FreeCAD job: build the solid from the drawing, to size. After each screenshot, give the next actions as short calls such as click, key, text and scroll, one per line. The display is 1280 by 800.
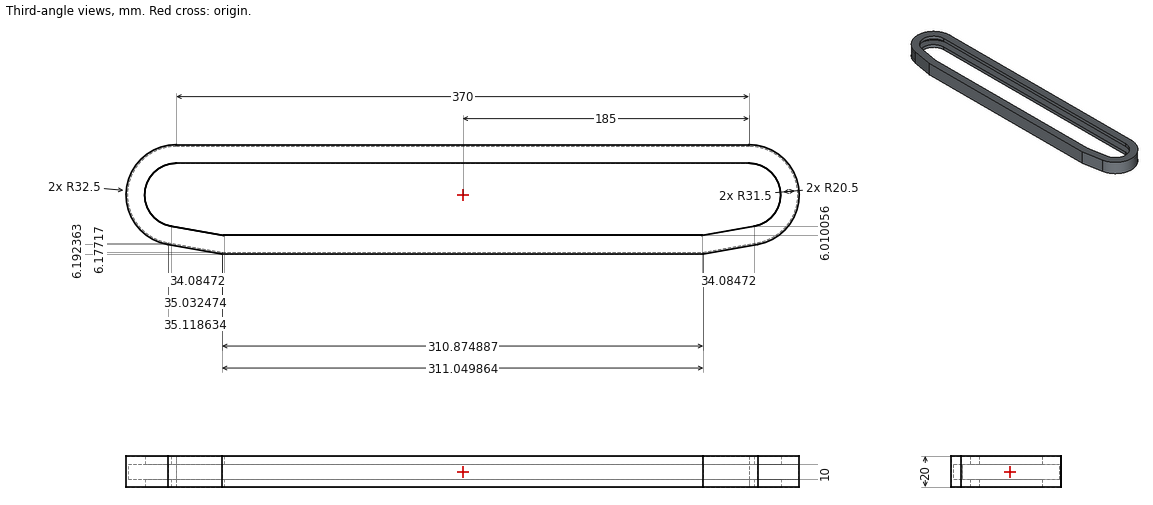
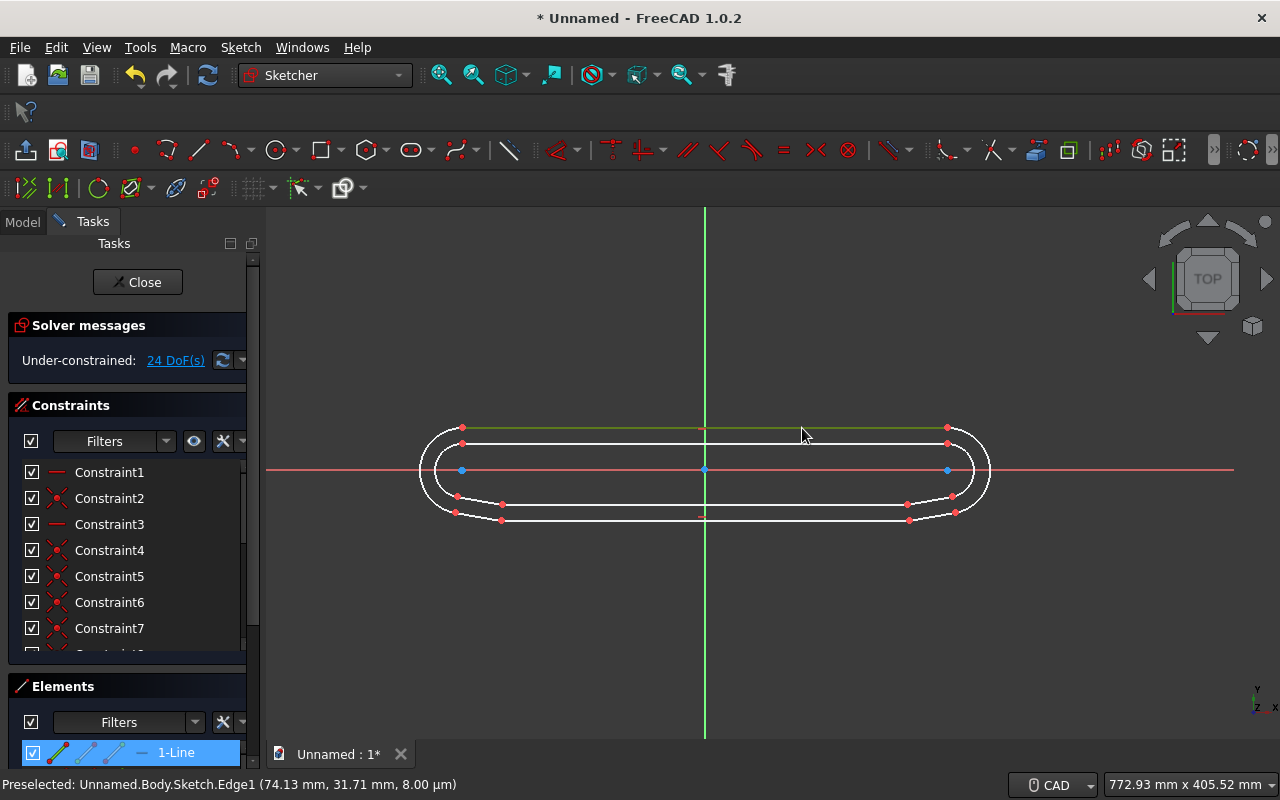
click(429, 444)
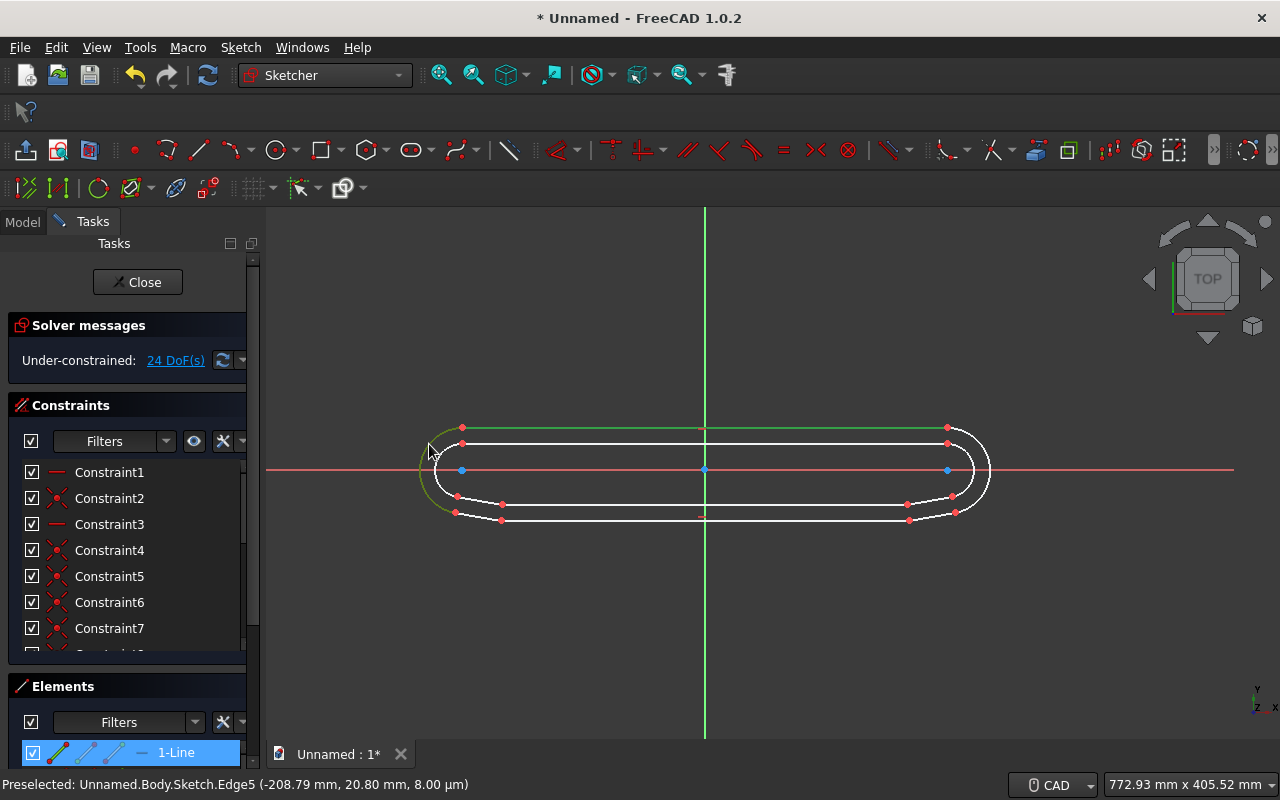
key(t)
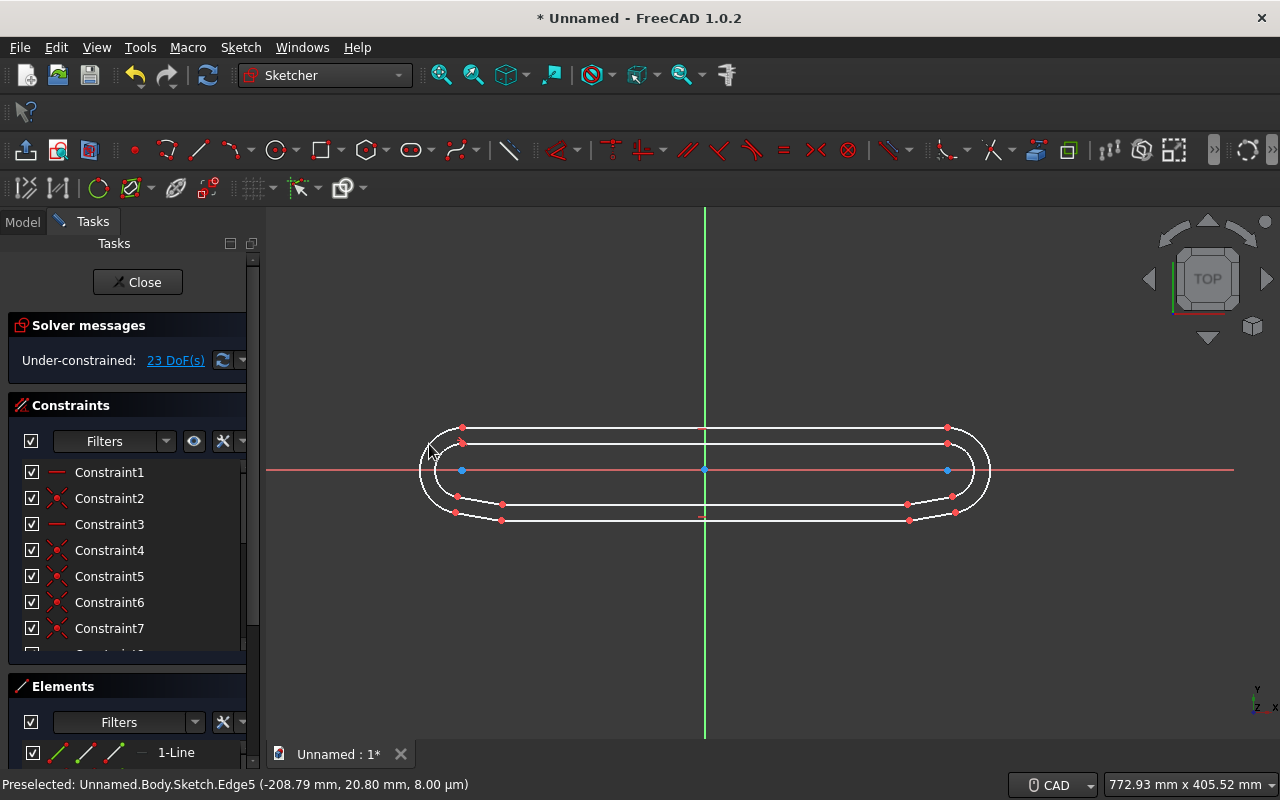
click(802, 428)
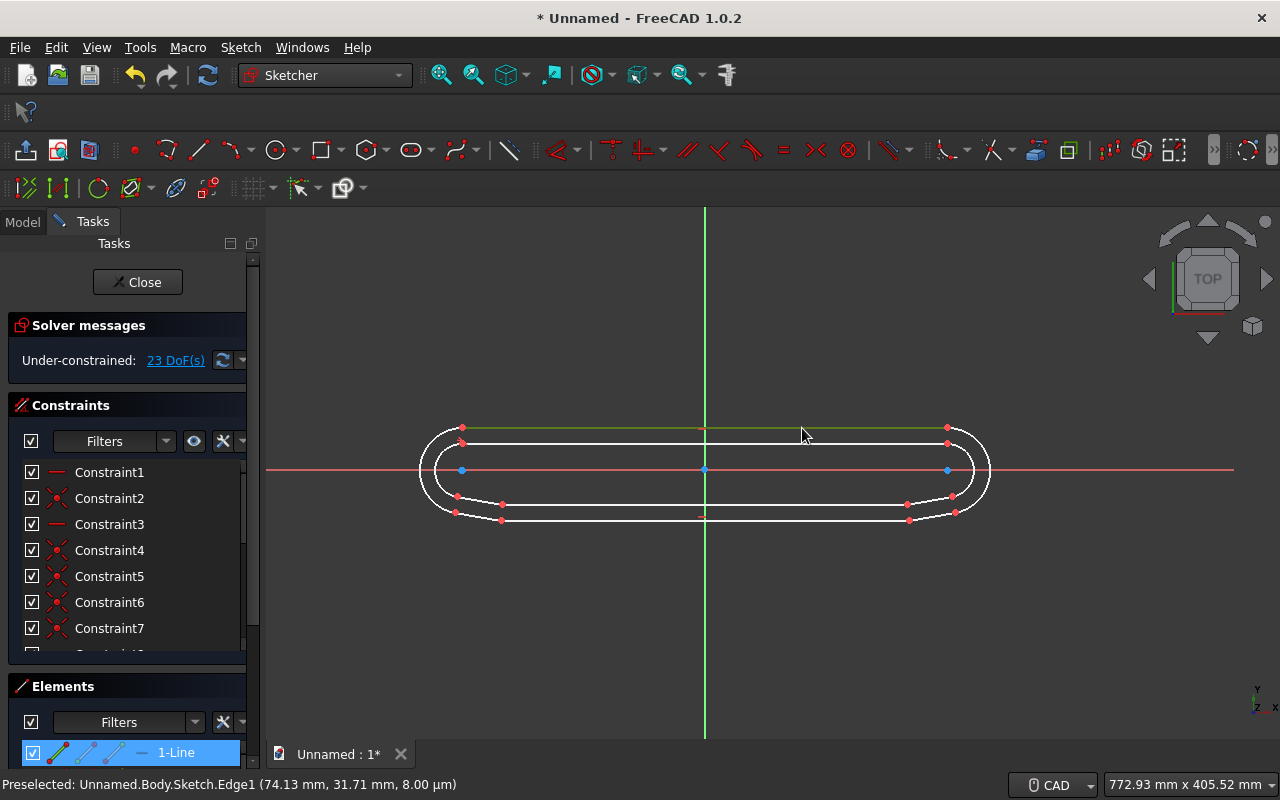
click(985, 491)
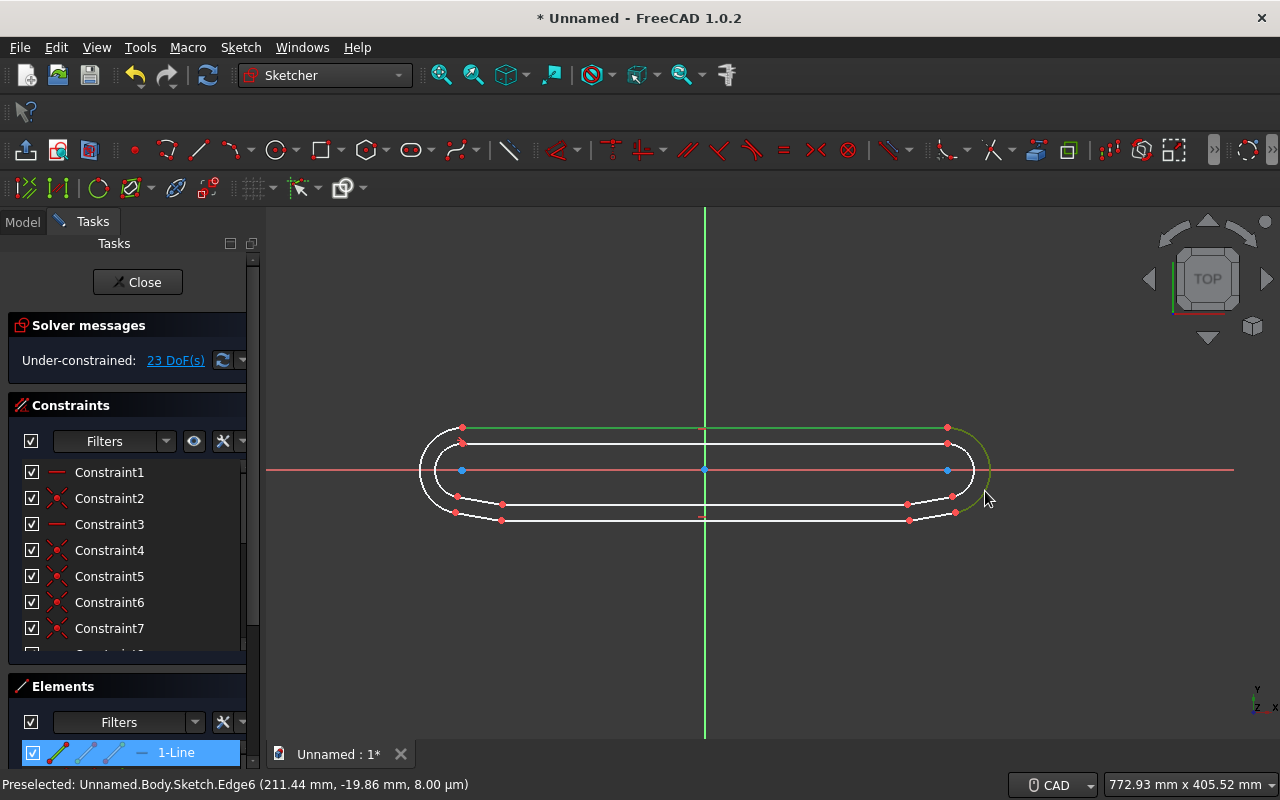
click(752, 150)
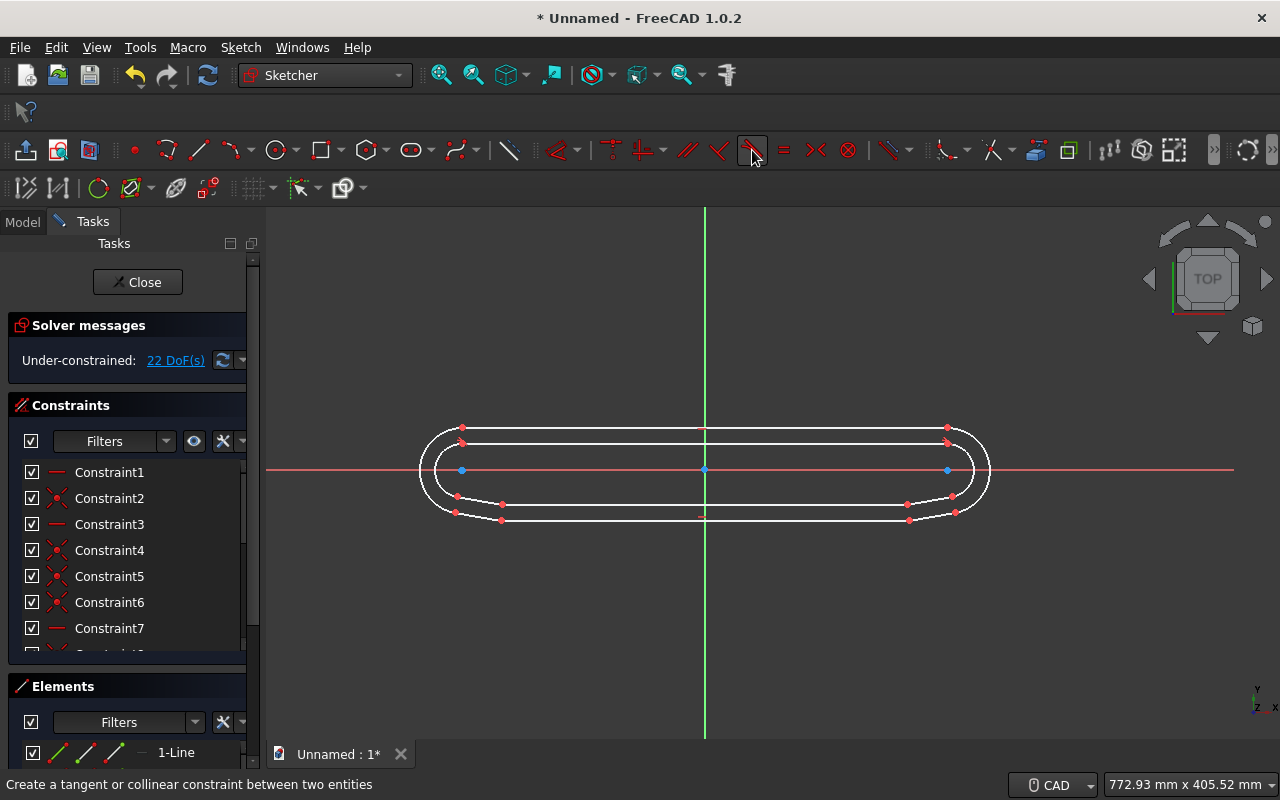
click(469, 515)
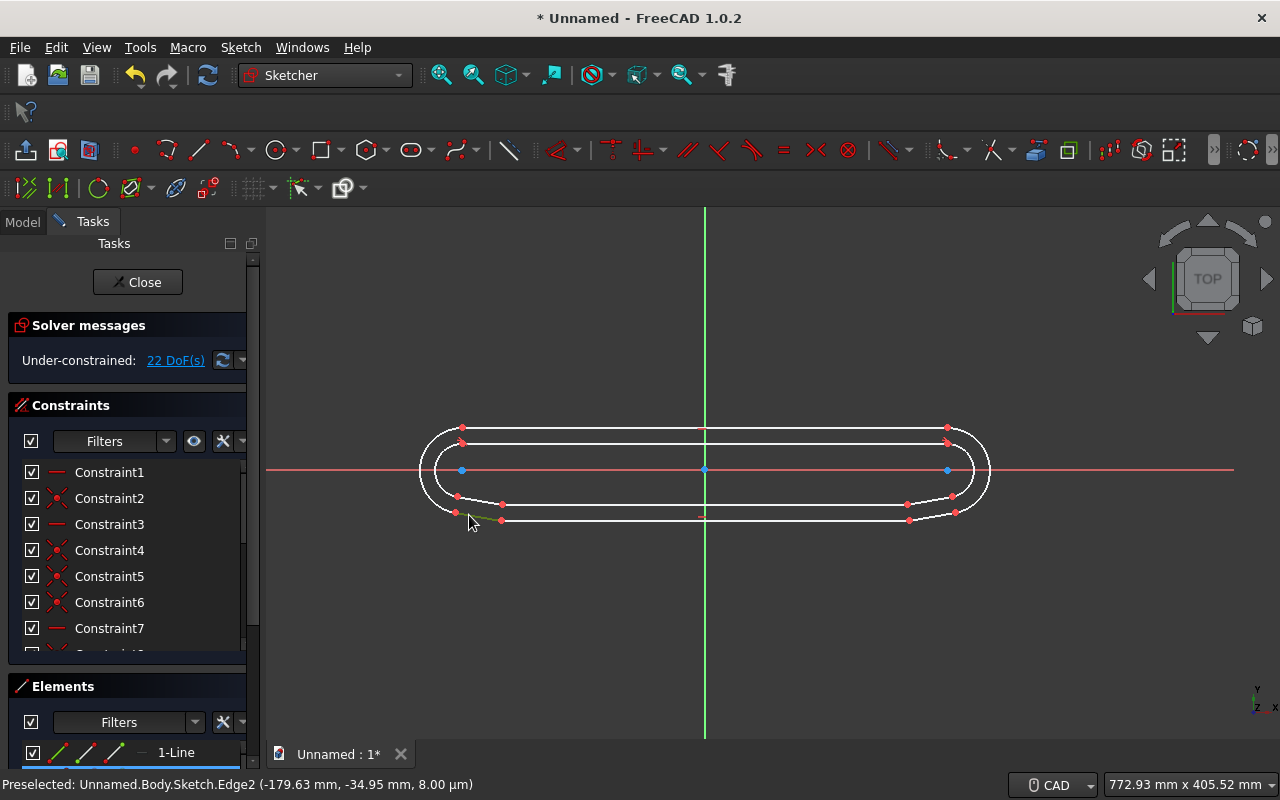
click(430, 444)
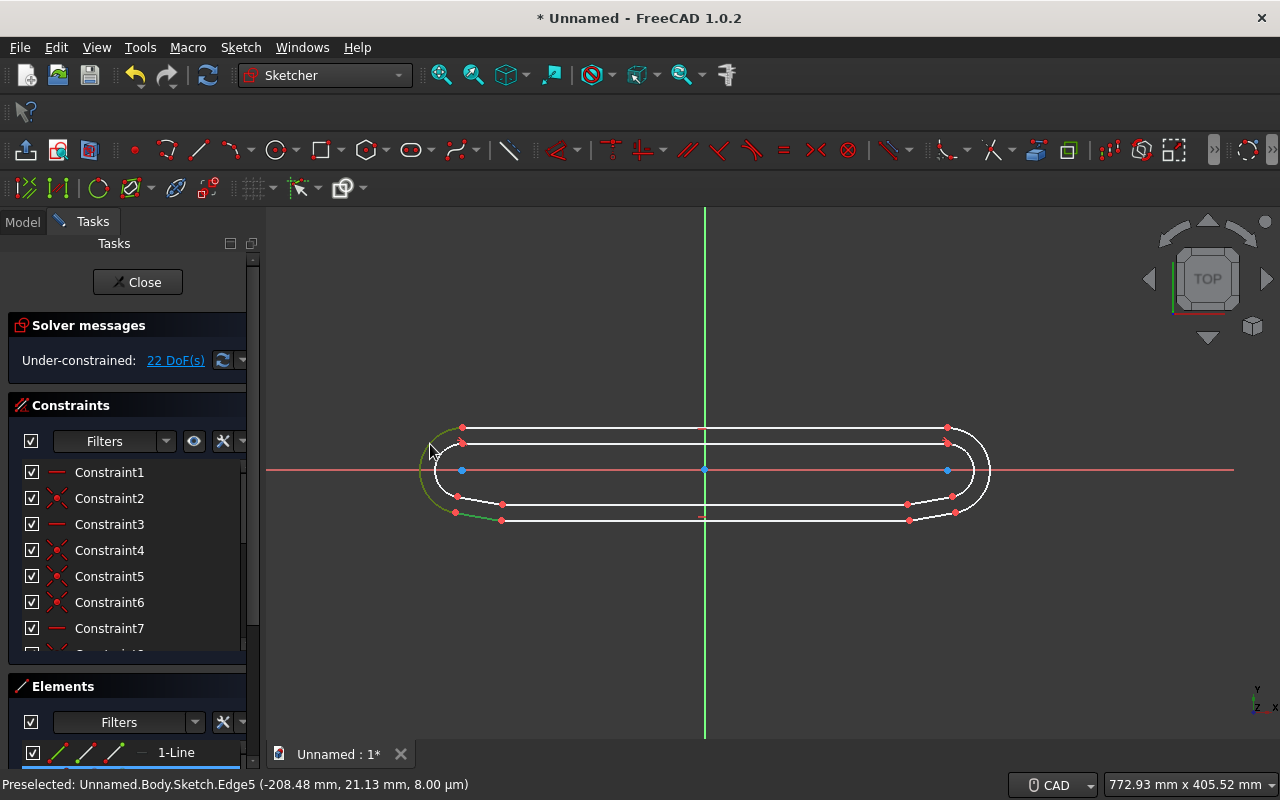
key(t)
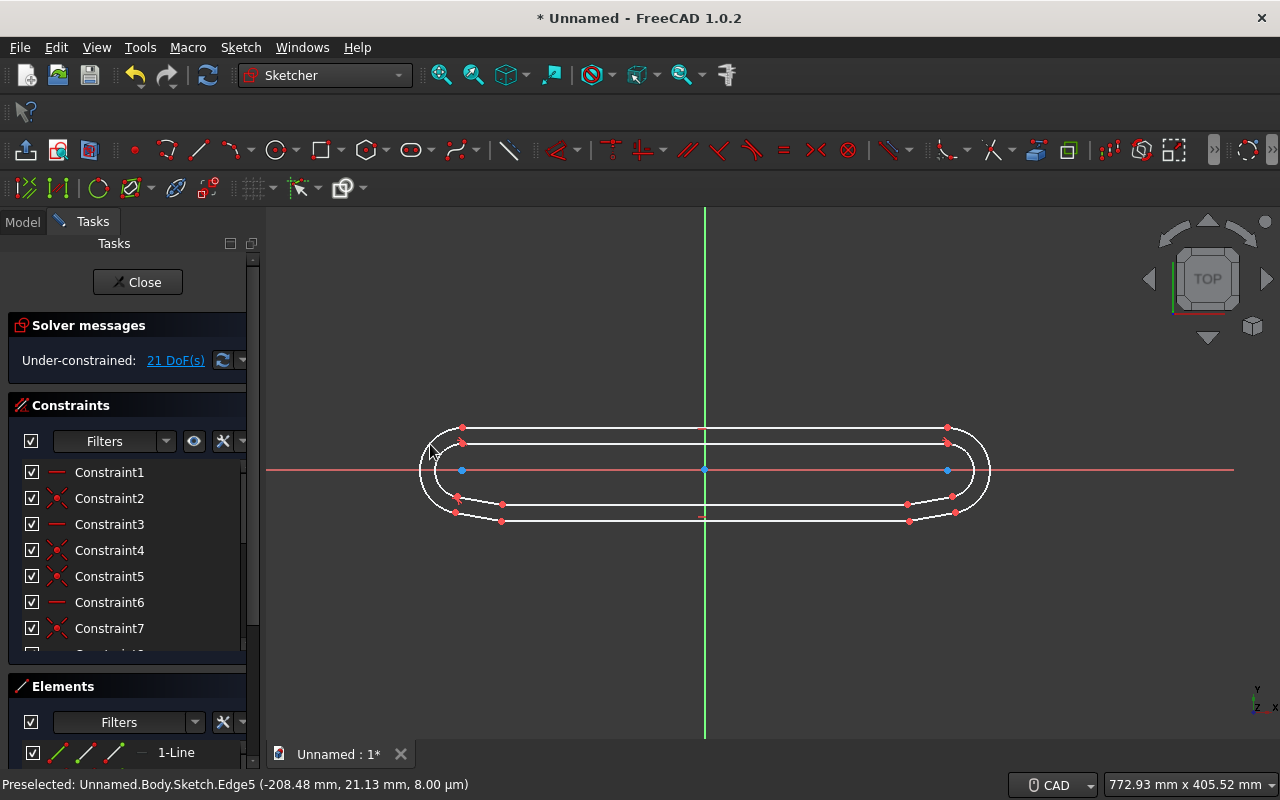
click(923, 519)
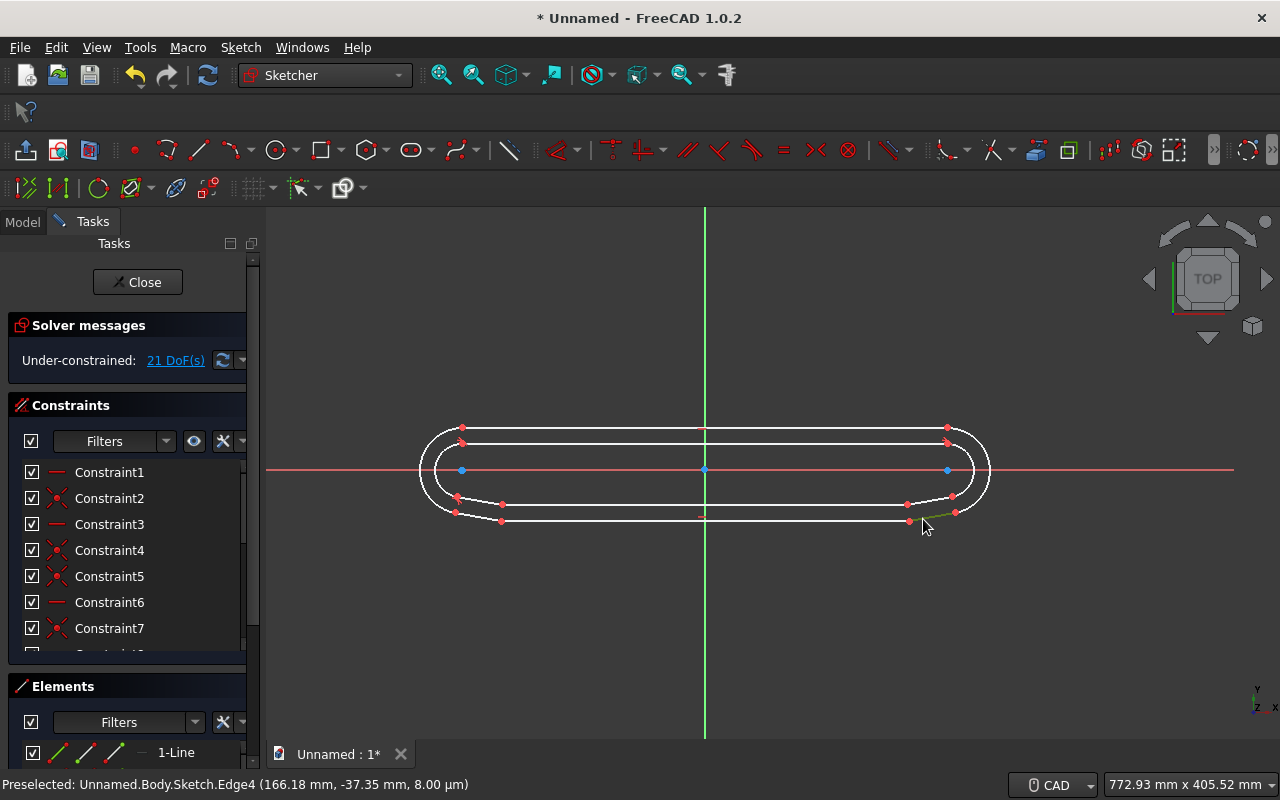
click(985, 491)